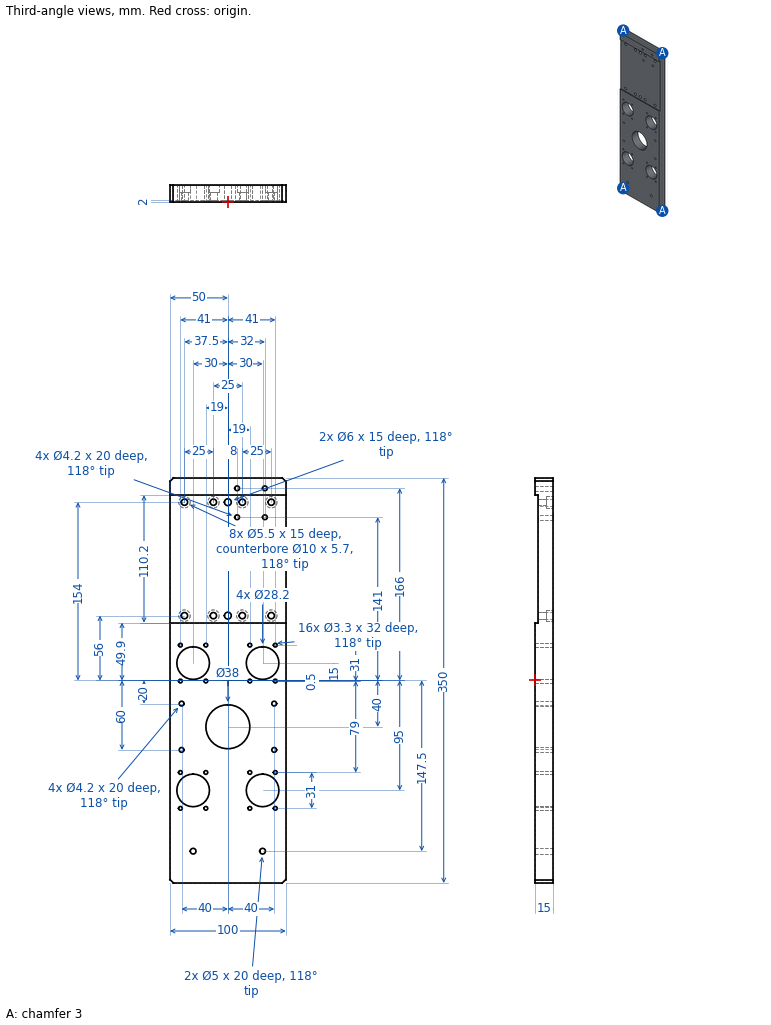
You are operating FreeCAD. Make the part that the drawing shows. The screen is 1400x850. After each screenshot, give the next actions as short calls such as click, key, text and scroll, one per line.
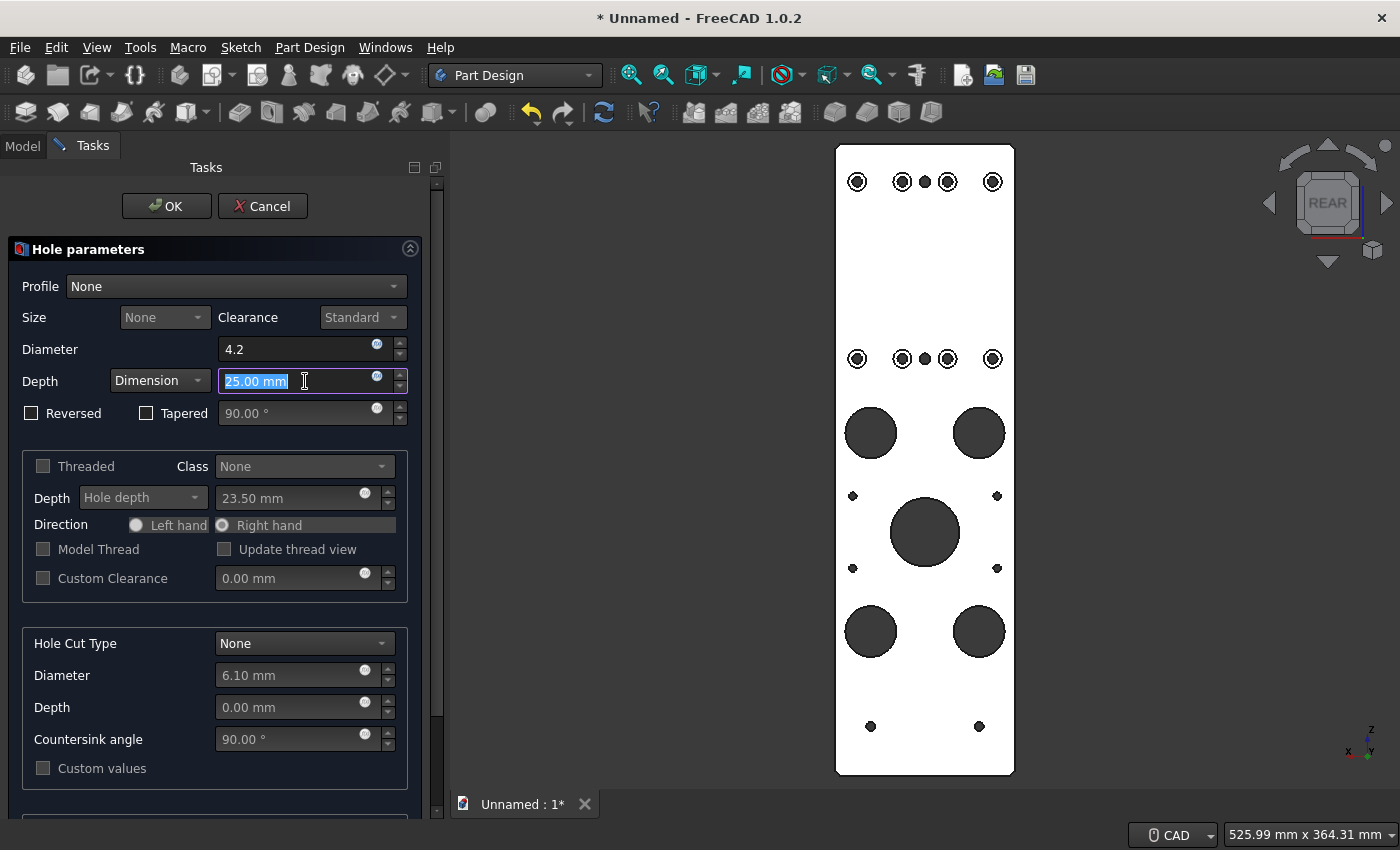
text(20)
key(Tab)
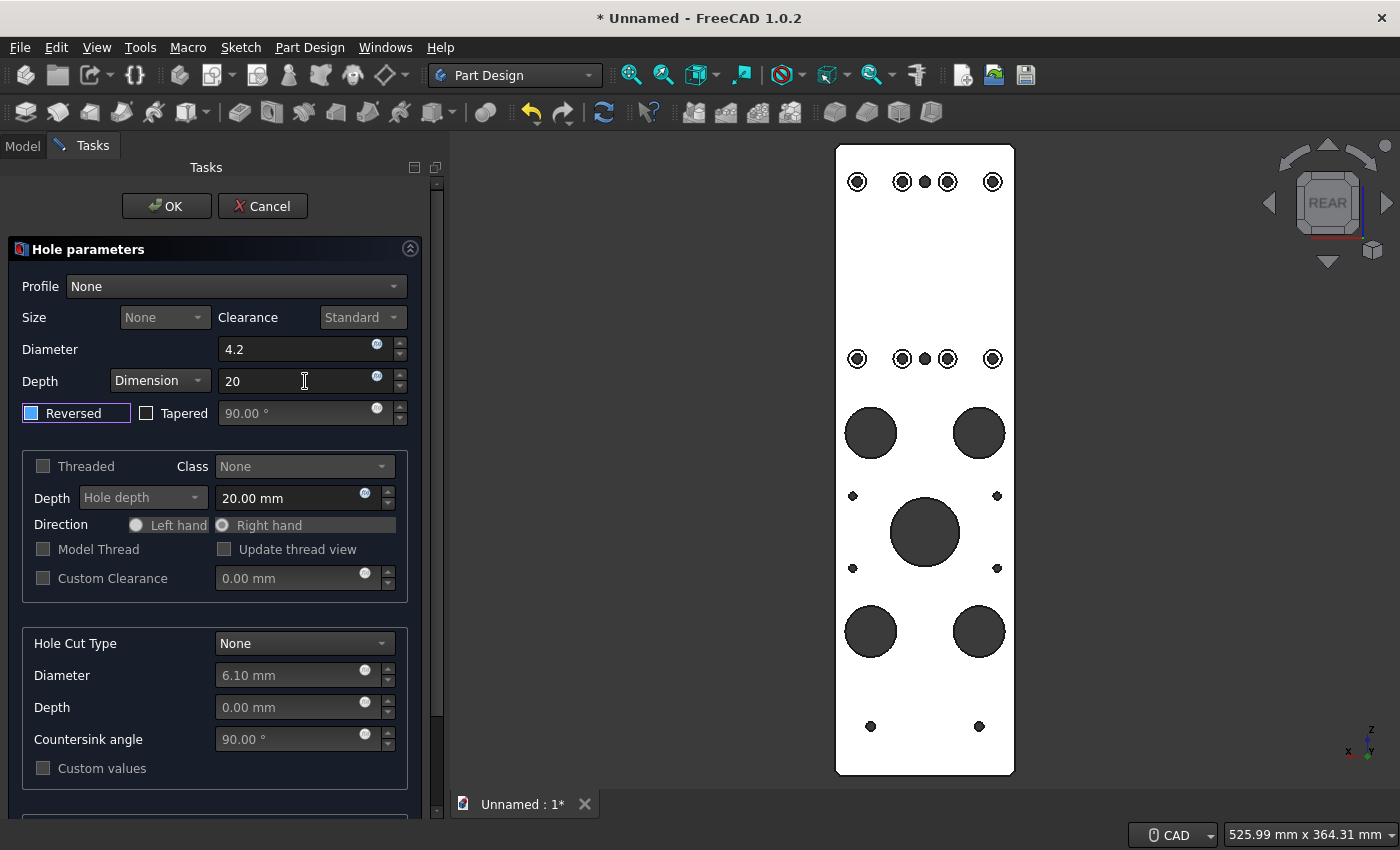
click(167, 206)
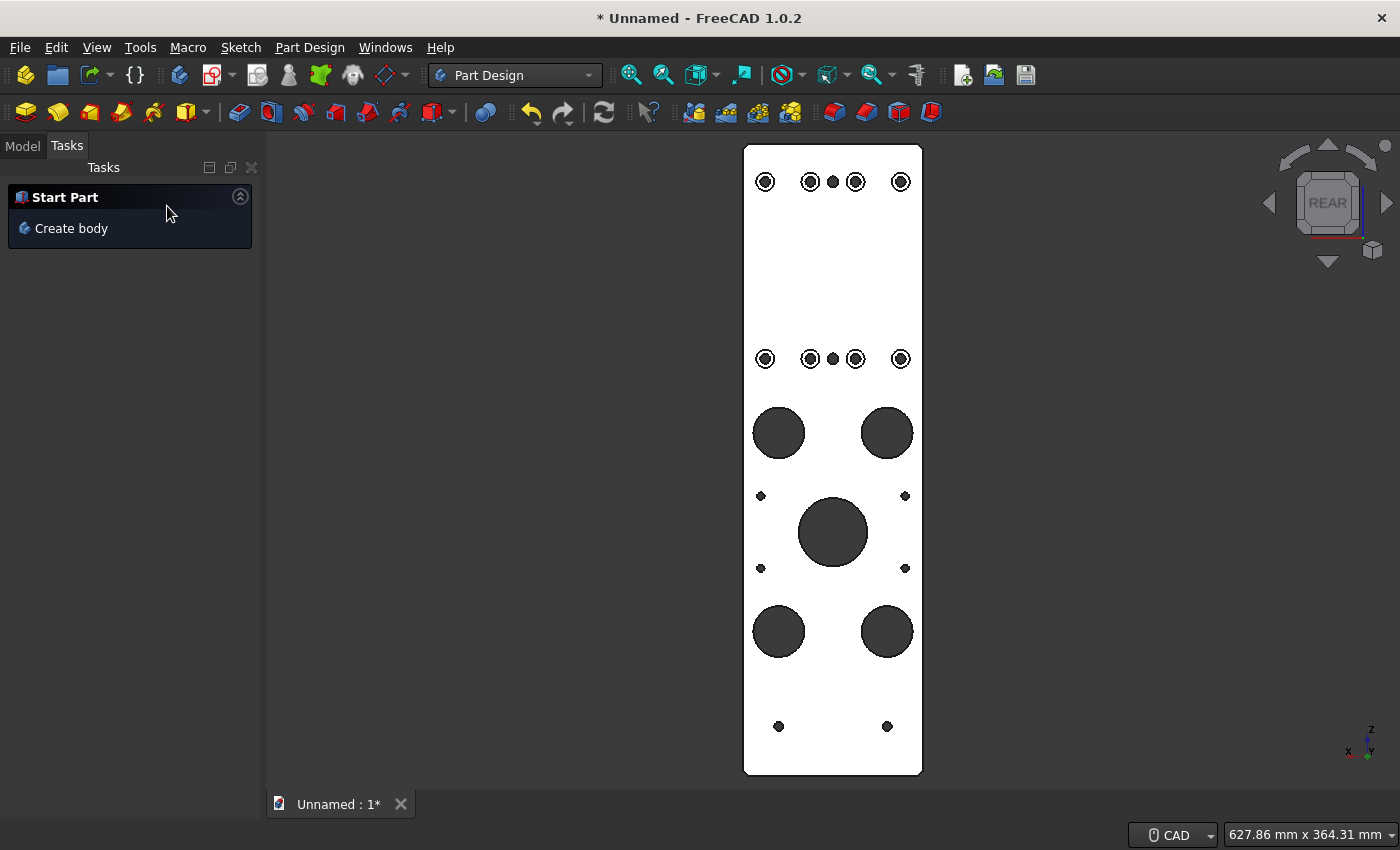
click(833, 278)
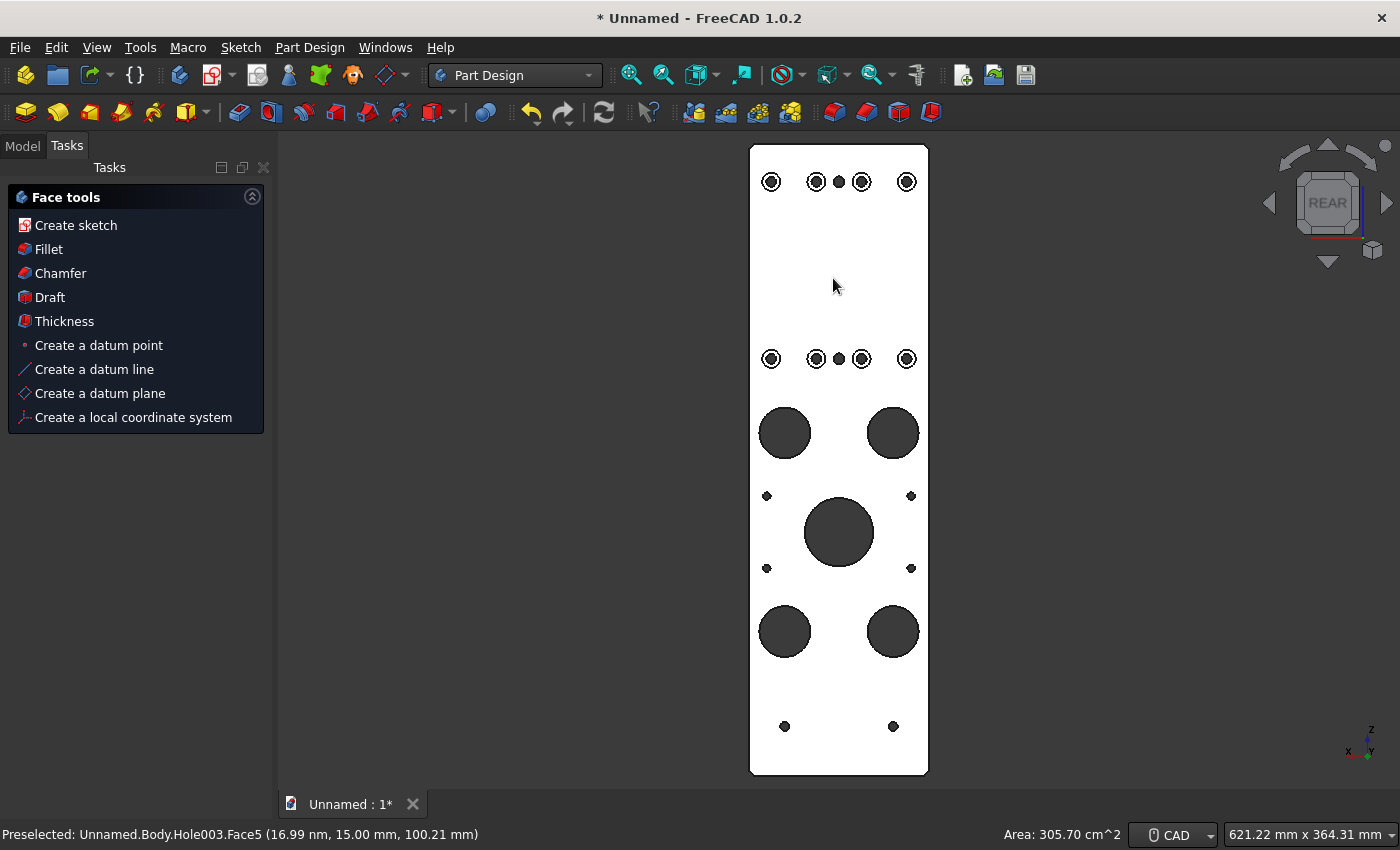
click(212, 76)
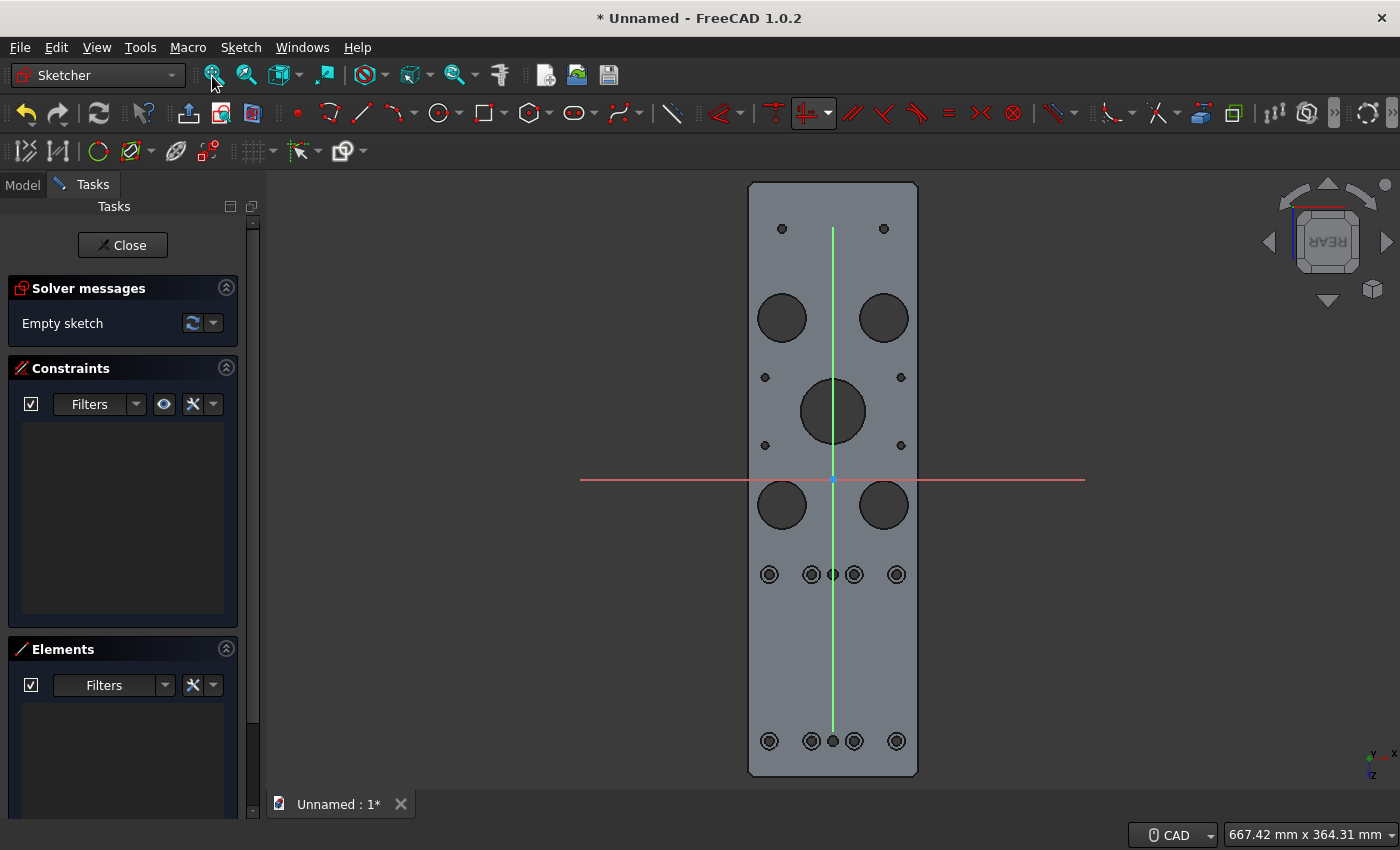
scroll(972, 273, up, 2)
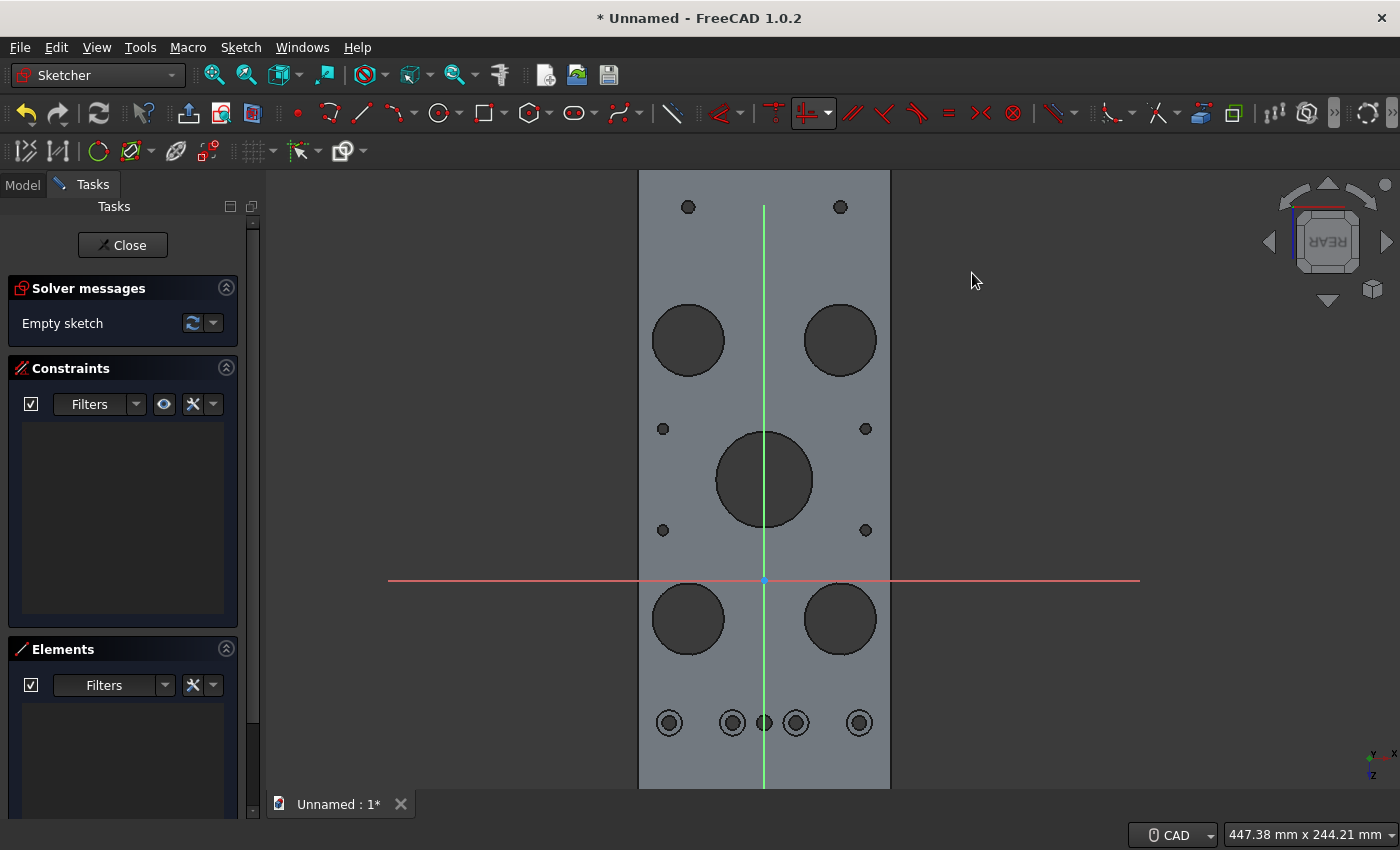
key(g)
key(c)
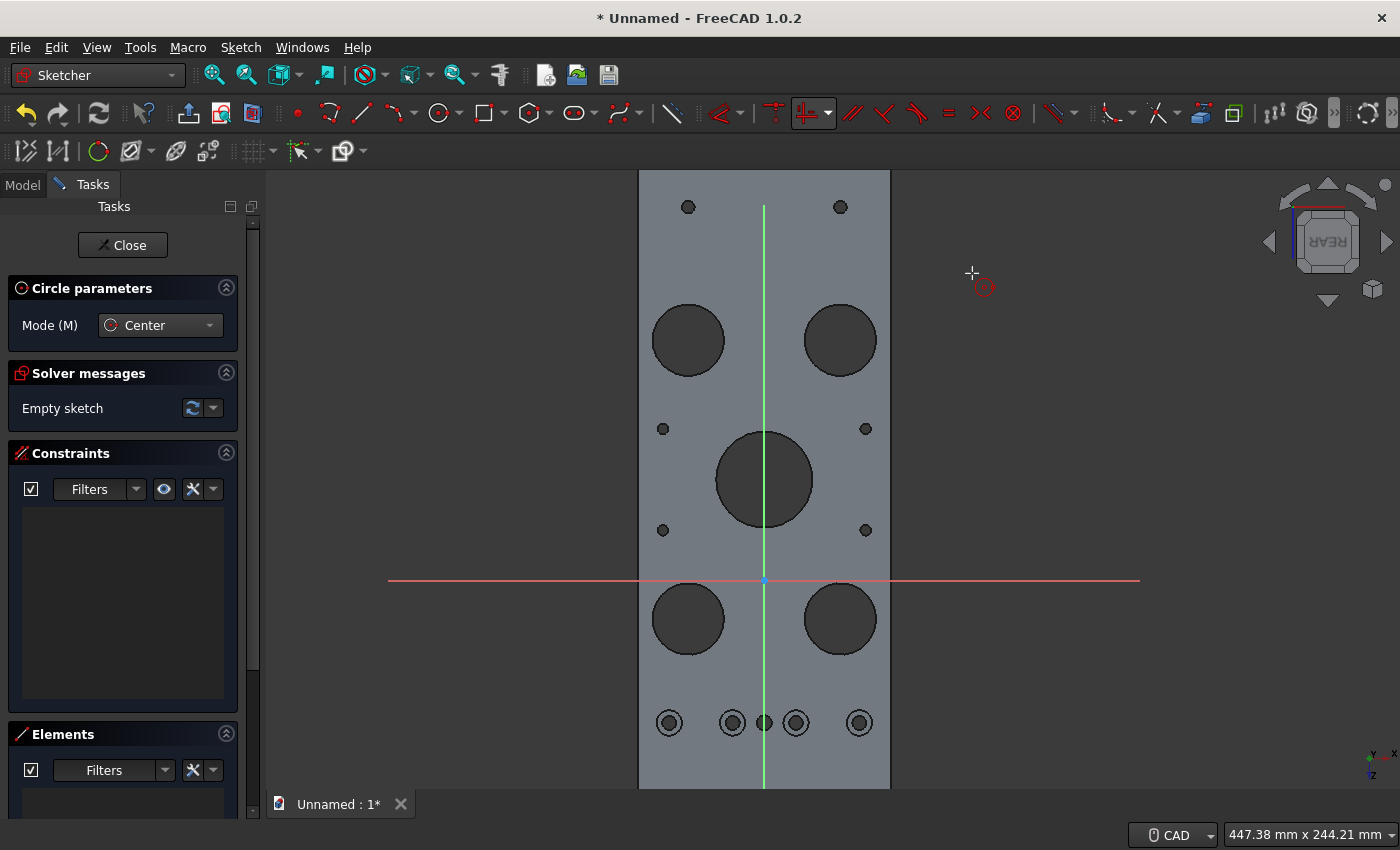
scroll(868, 658, up, 9)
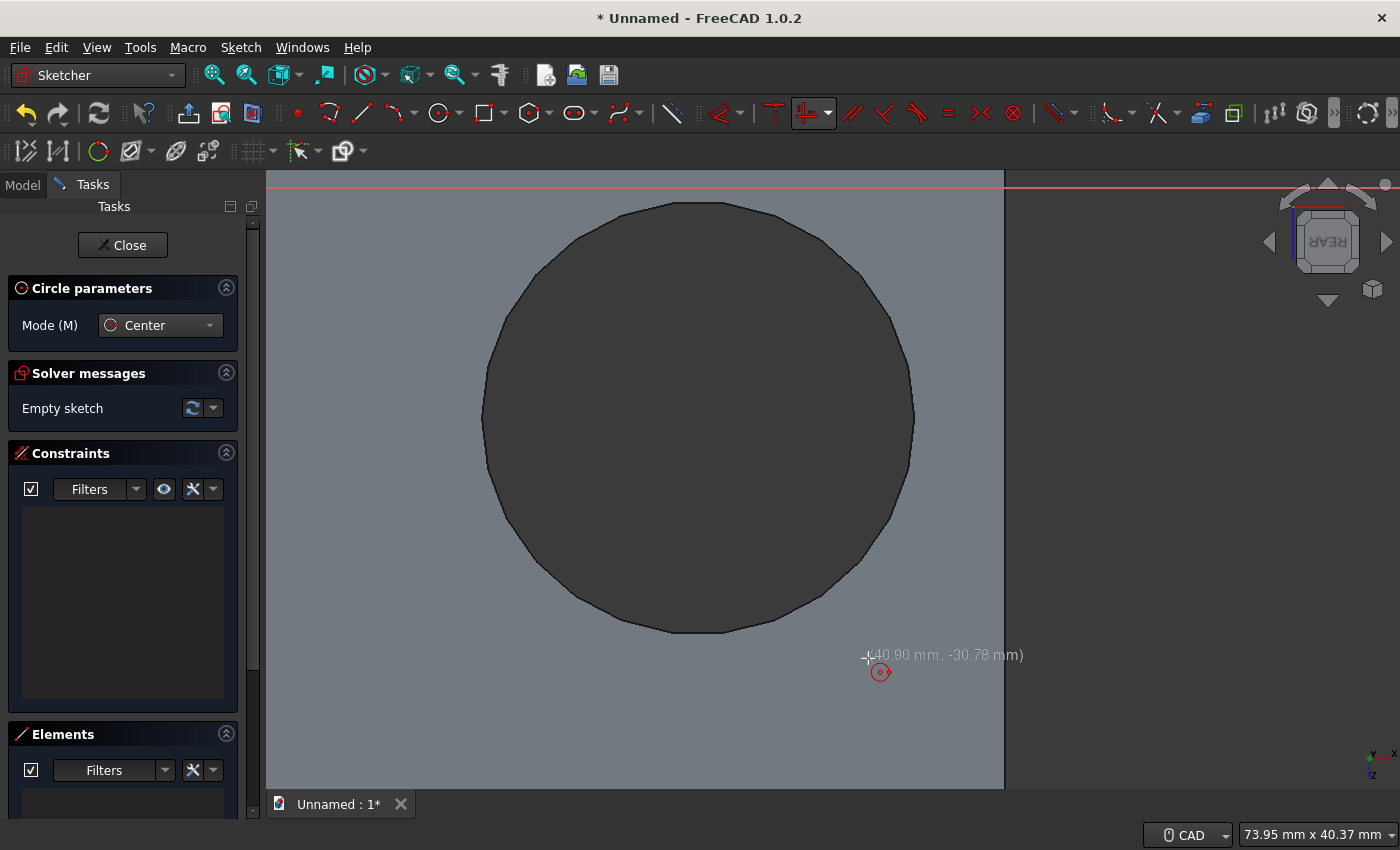
scroll(869, 659, down, 9)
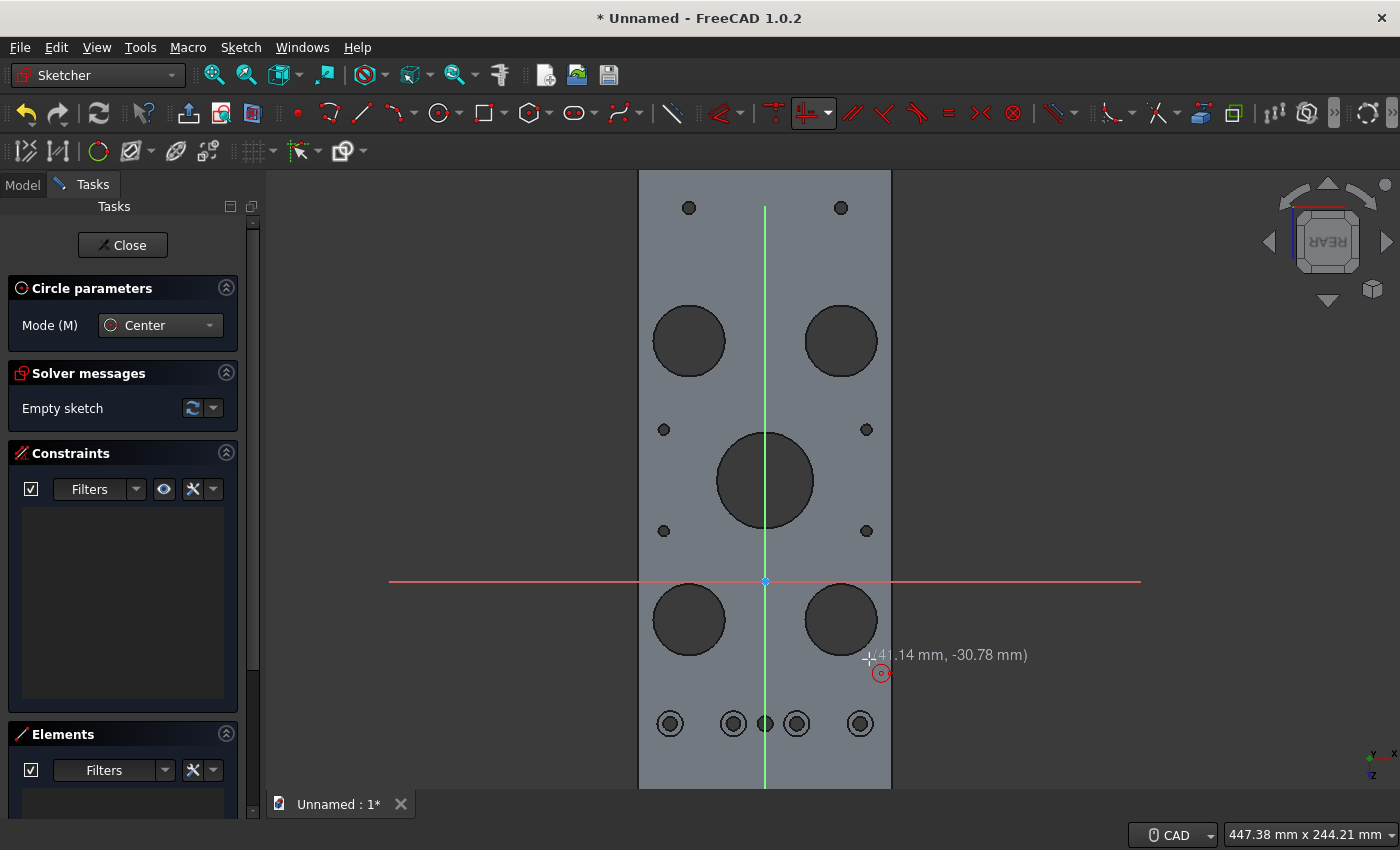
click(869, 659)